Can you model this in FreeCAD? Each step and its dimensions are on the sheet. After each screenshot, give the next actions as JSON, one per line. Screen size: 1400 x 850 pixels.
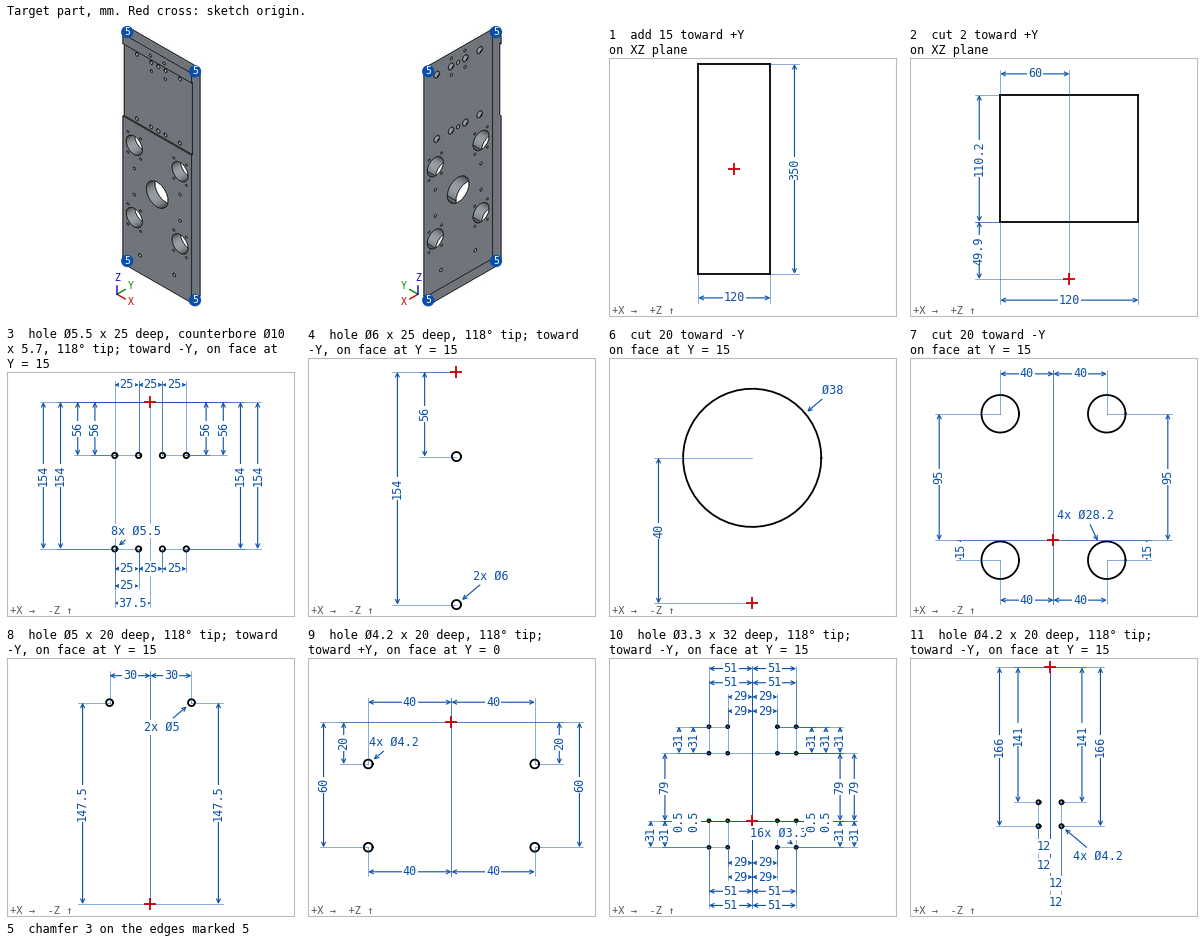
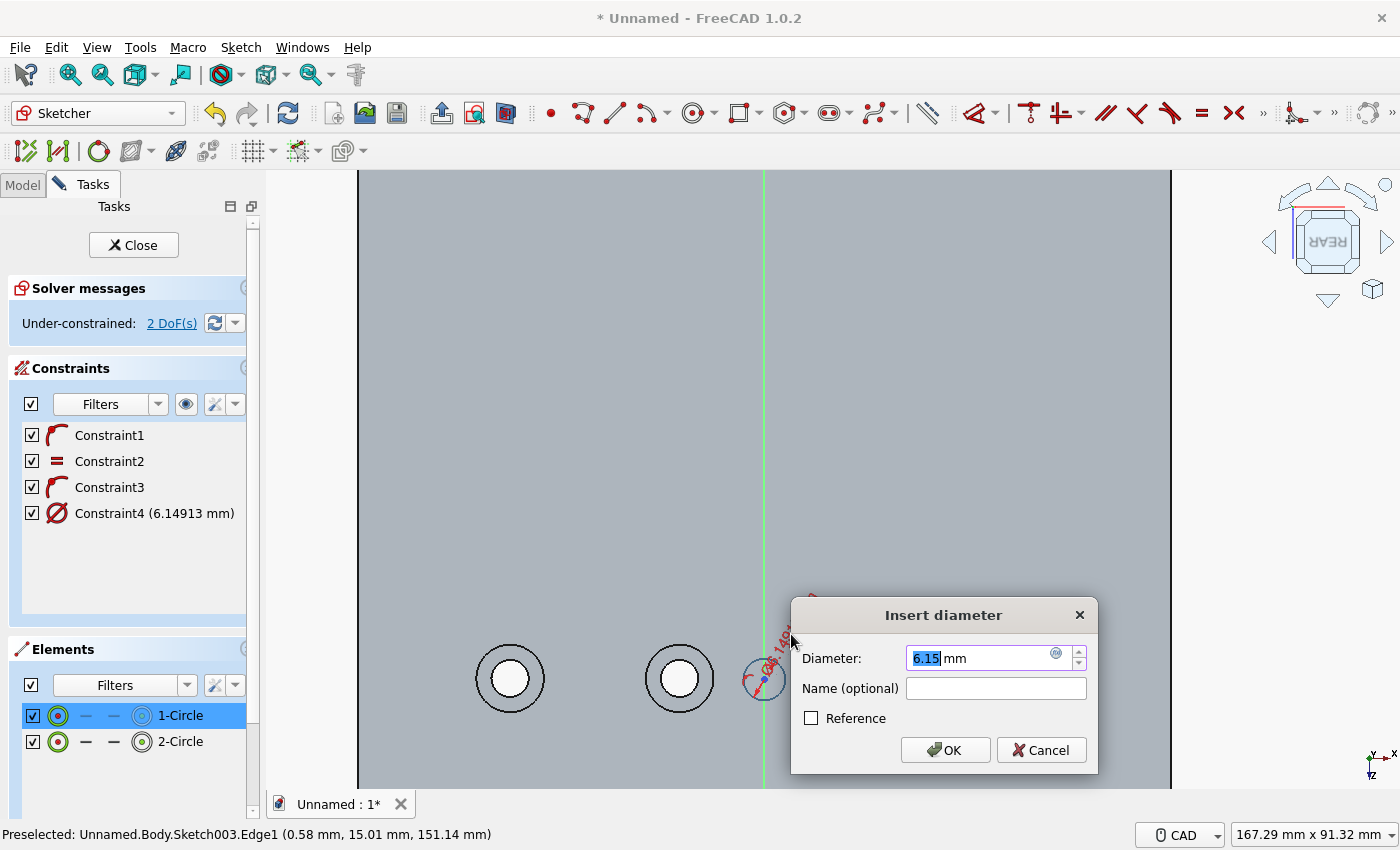
{"action": "type", "text": "6"}
{"action": "key", "text": "Return"}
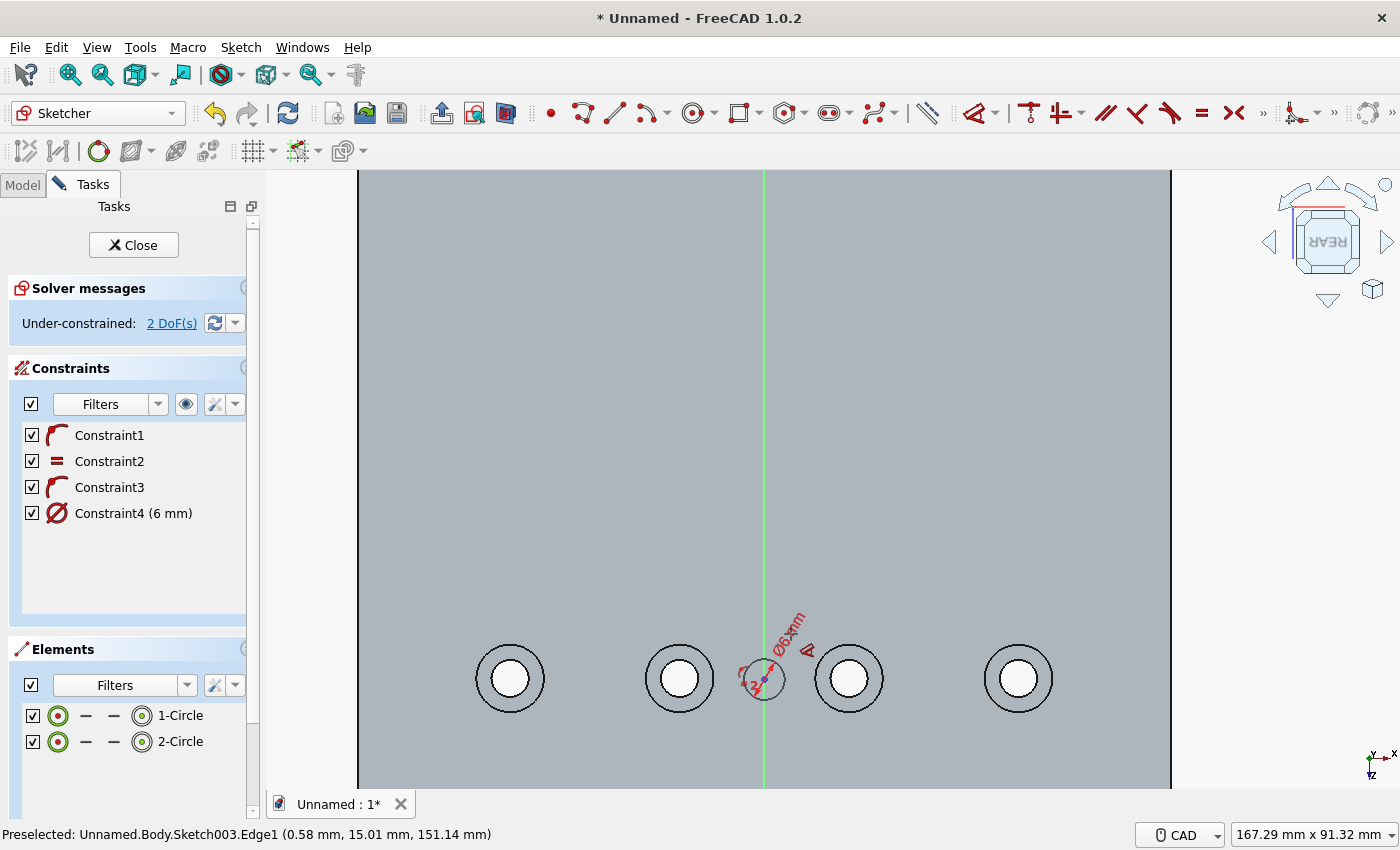
{"action": "scroll", "coordinate": [765, 662], "scroll_direction": "down", "scroll_amount": 5}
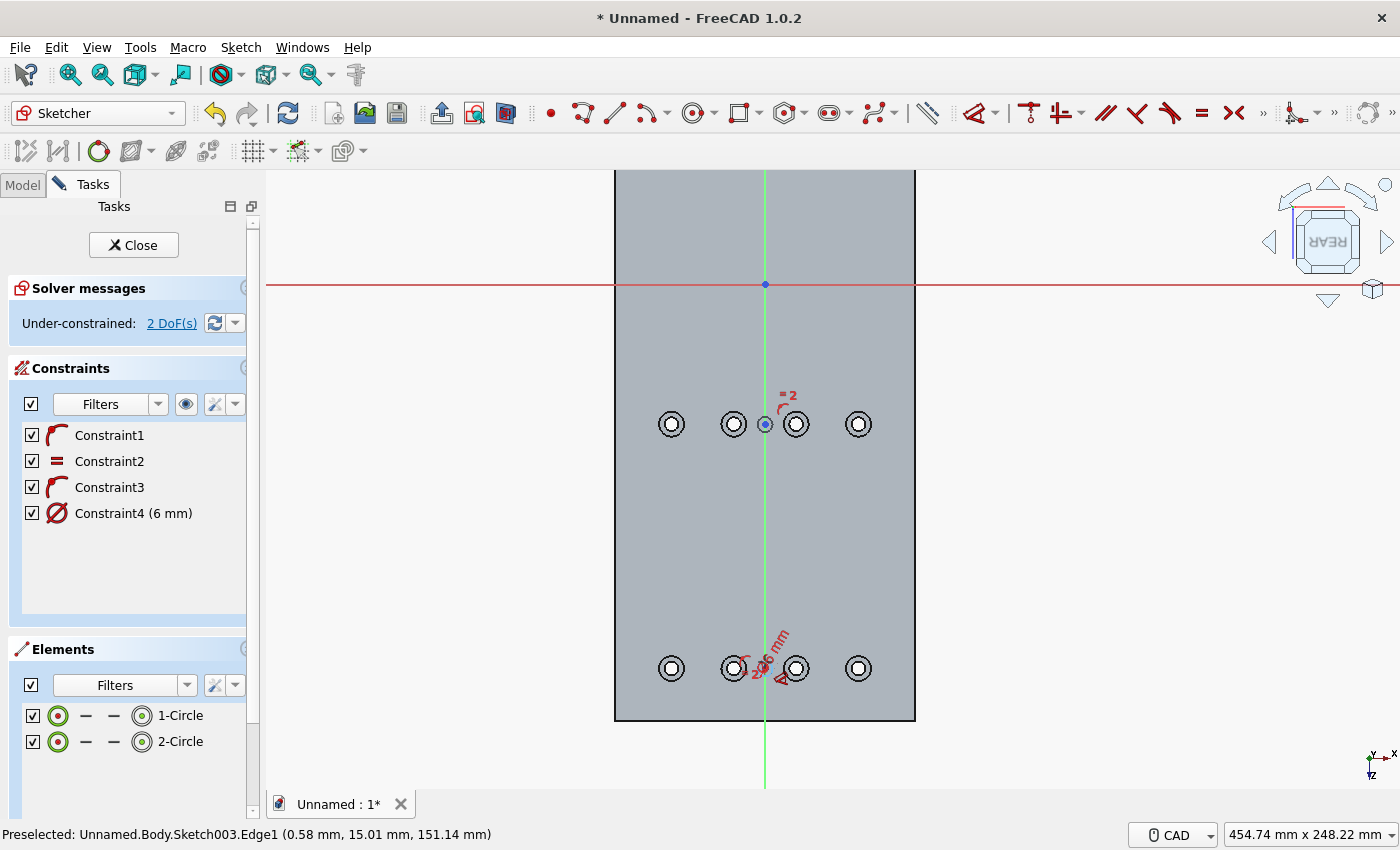
{"action": "left_click", "coordinate": [765, 425]}
{"action": "left_click", "coordinate": [799, 355]}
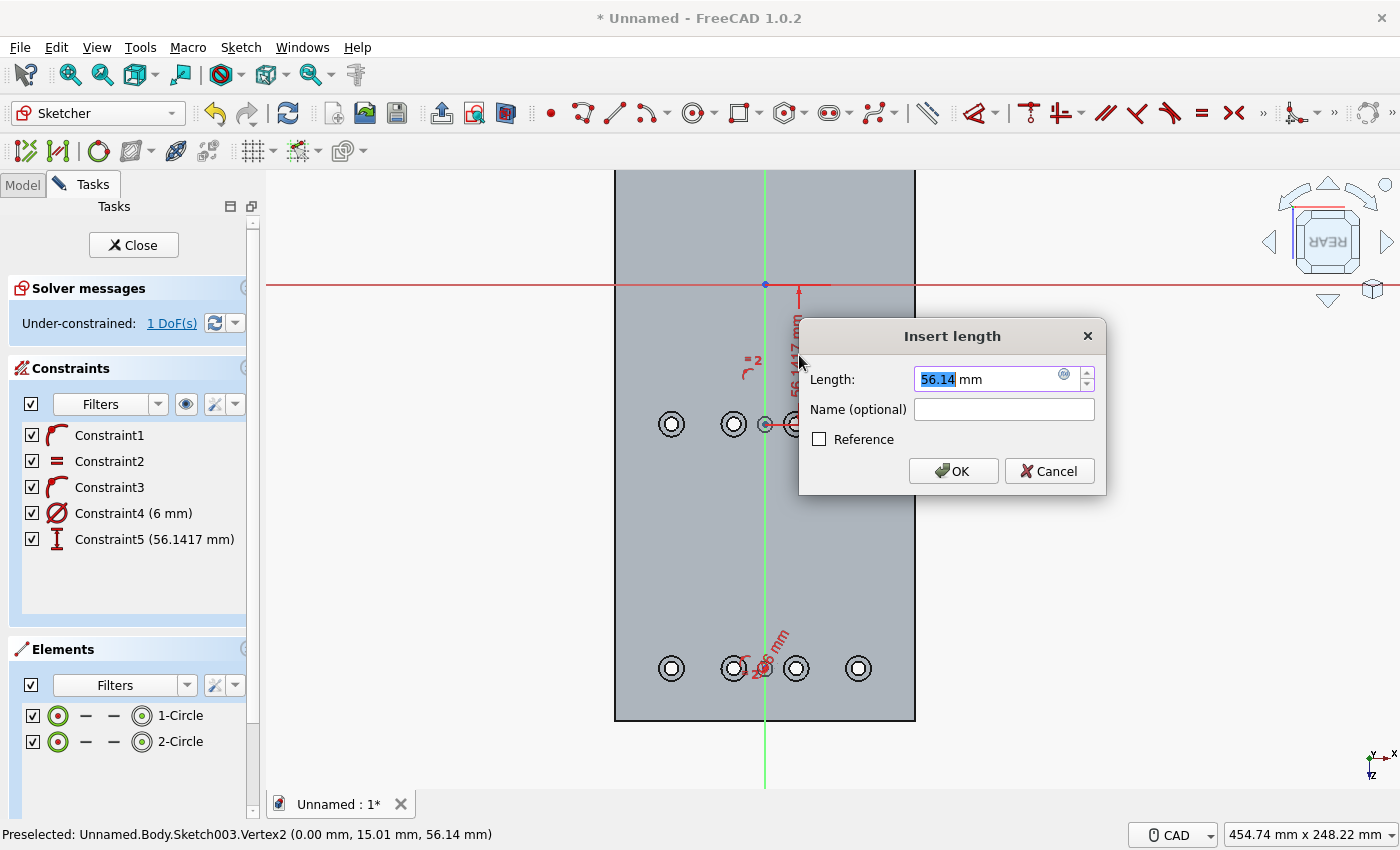
{"action": "type", "text": "56"}
{"action": "key", "text": "Return"}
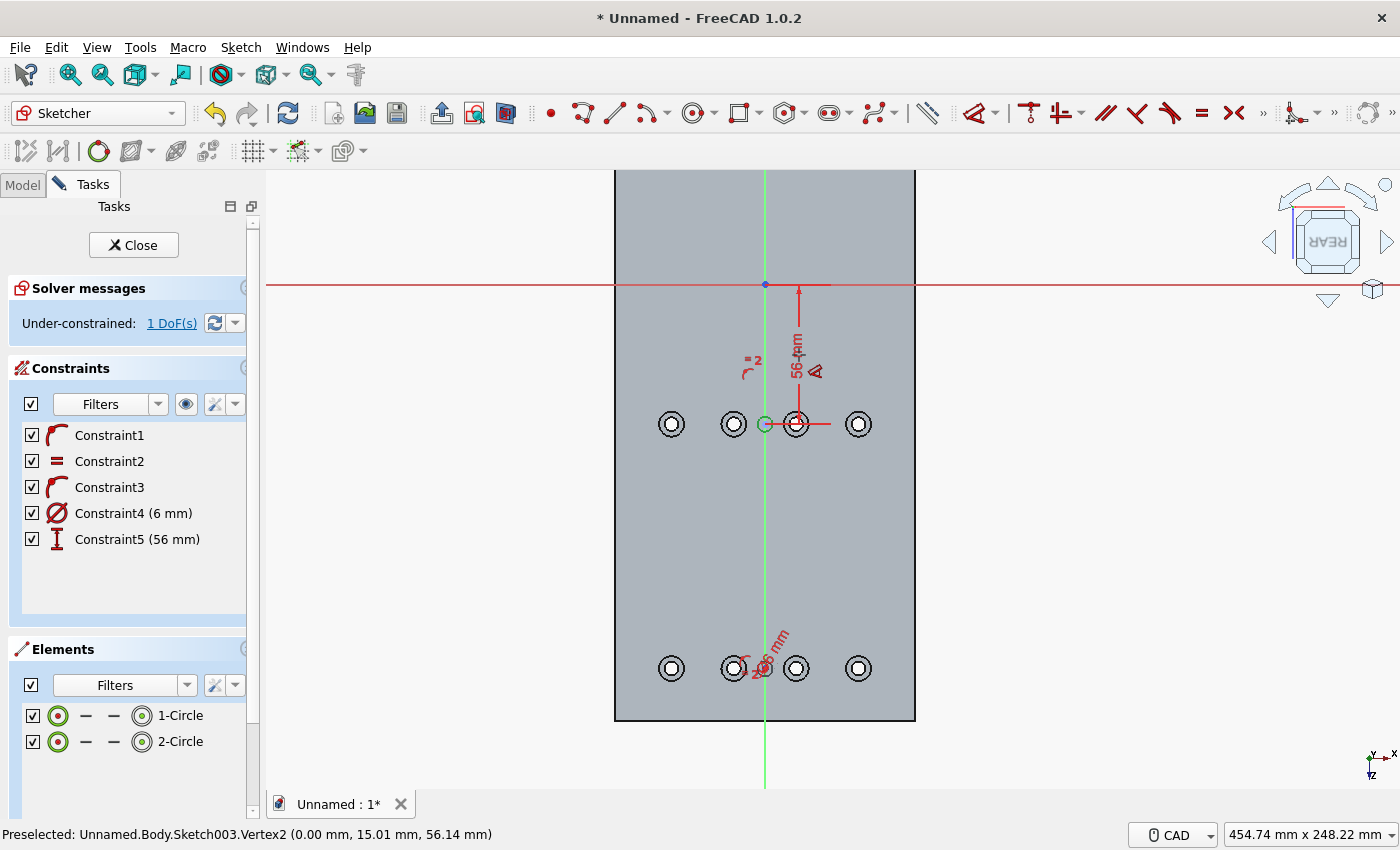
{"action": "left_click", "coordinate": [765, 669]}
{"action": "left_click", "coordinate": [799, 477]}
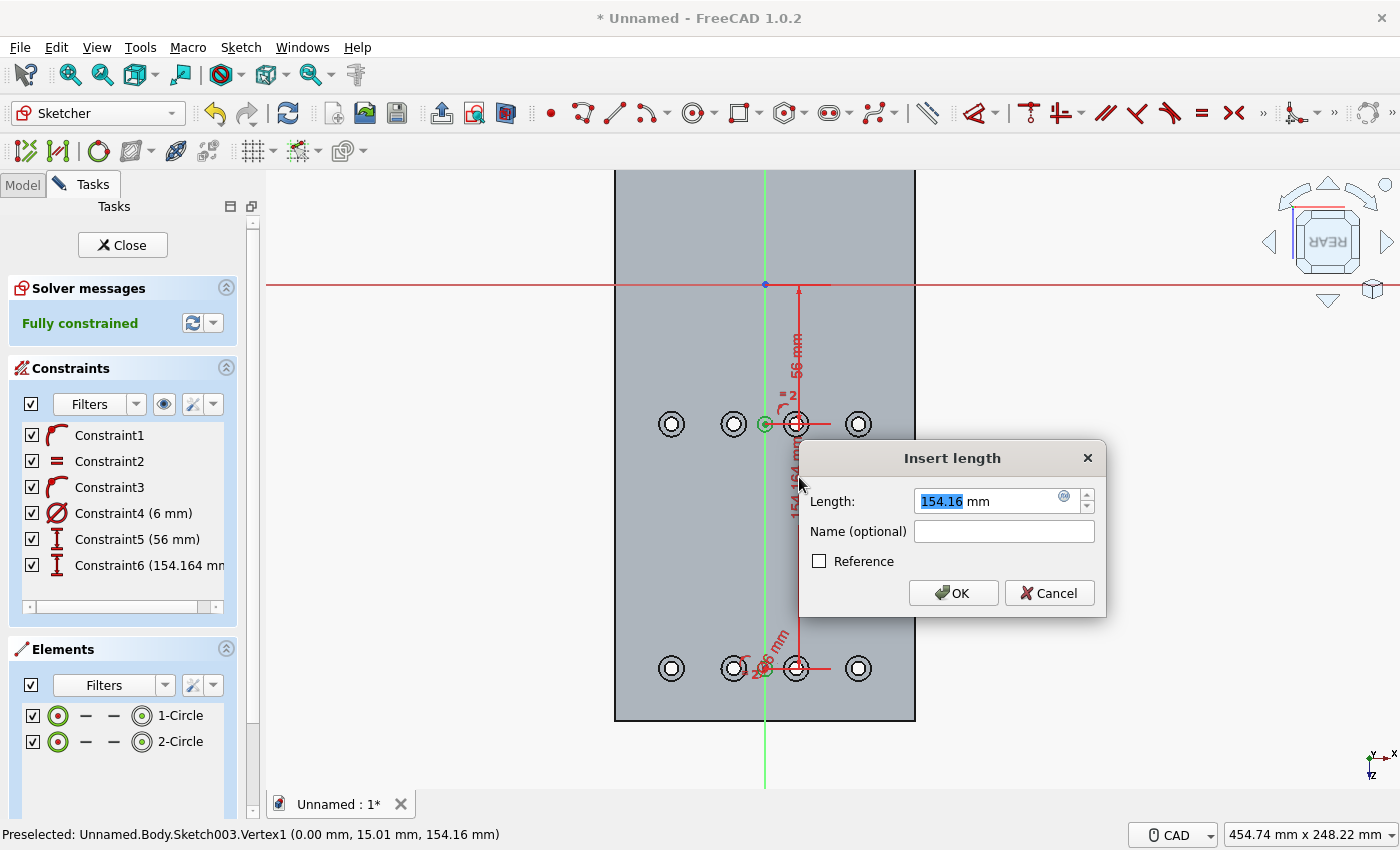
{"action": "type", "text": "154"}
{"action": "key", "text": "Return"}
{"action": "key", "text": "Escape"}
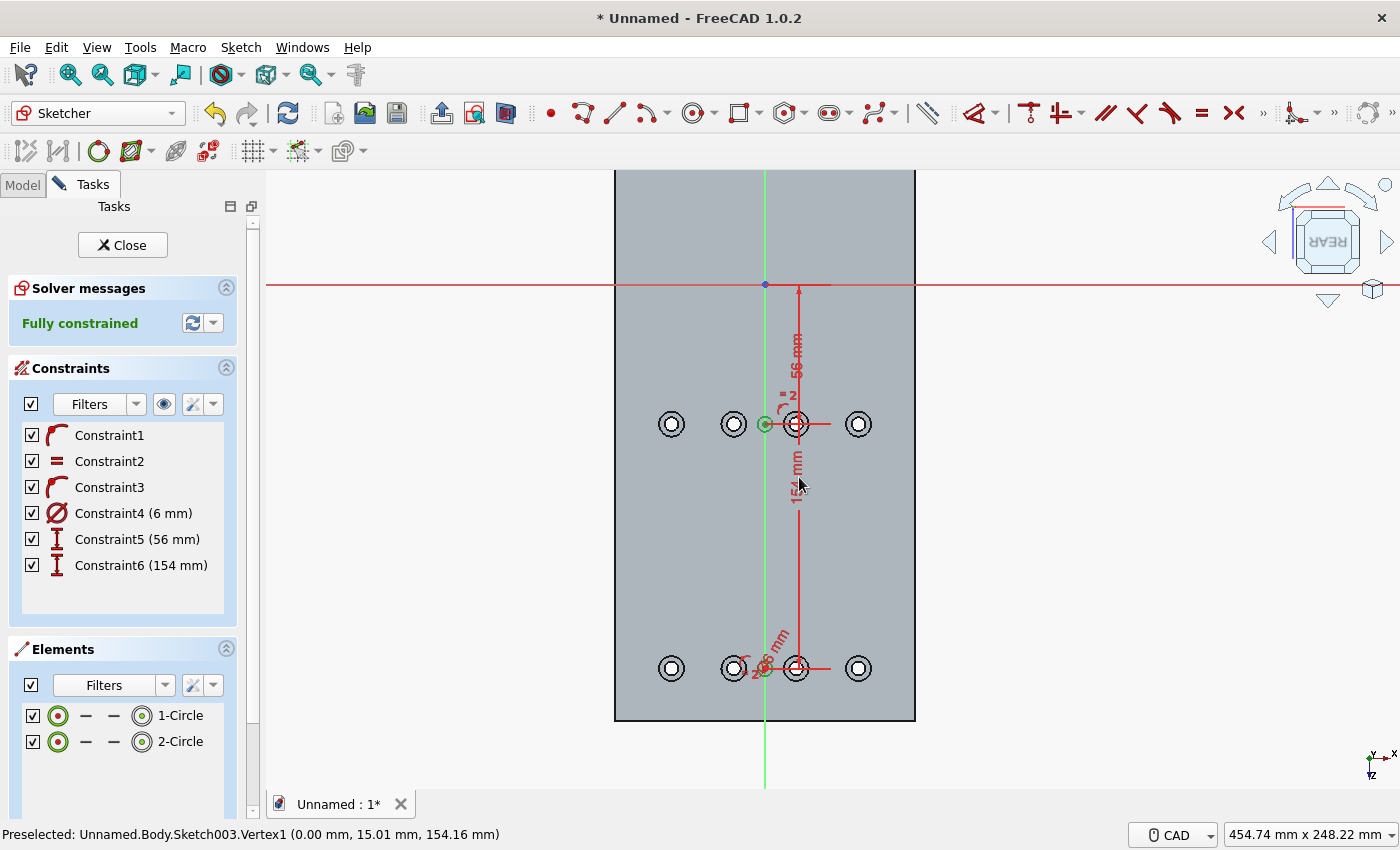
{"action": "left_click", "coordinate": [123, 245]}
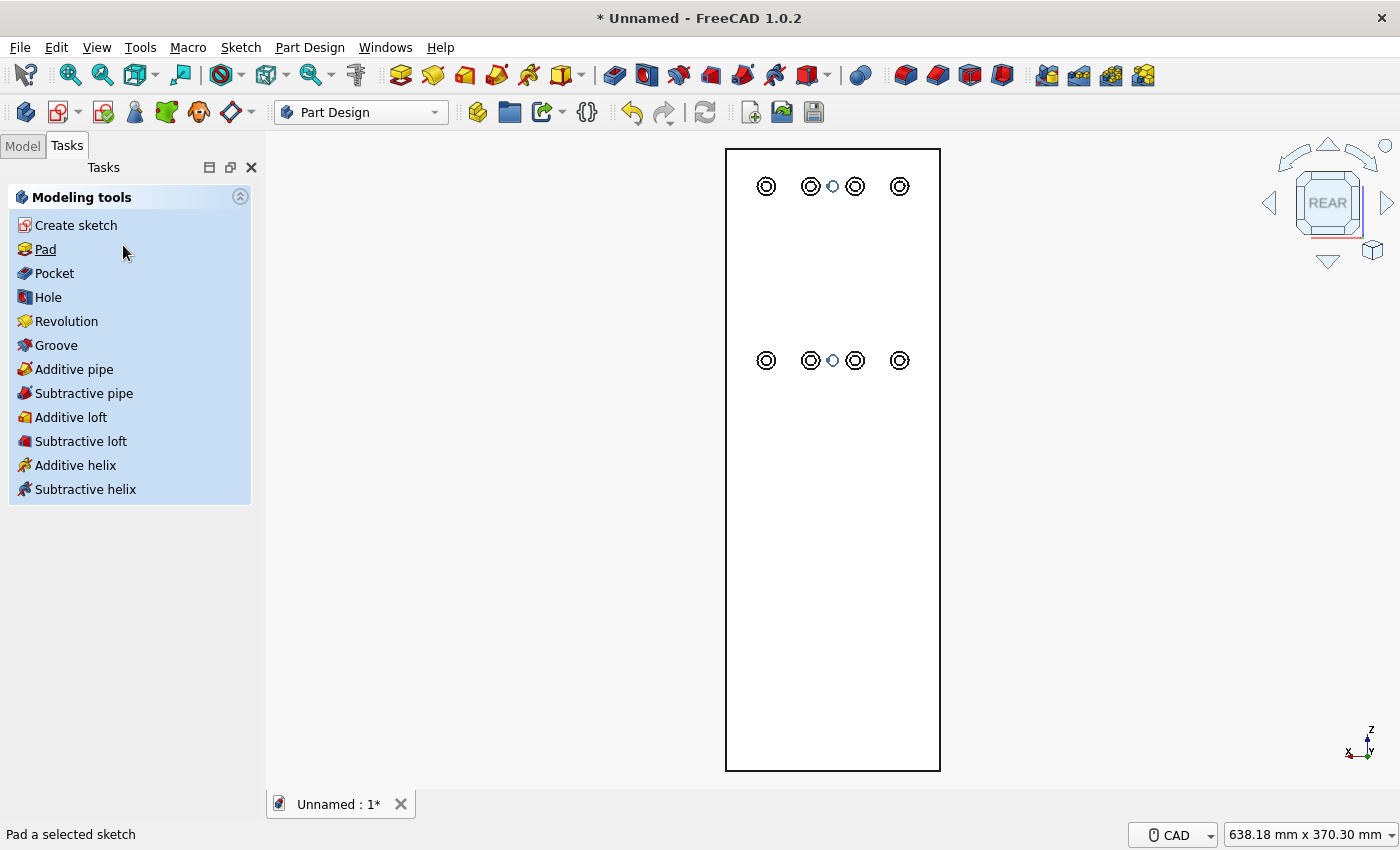
{"action": "left_click", "coordinate": [648, 76]}